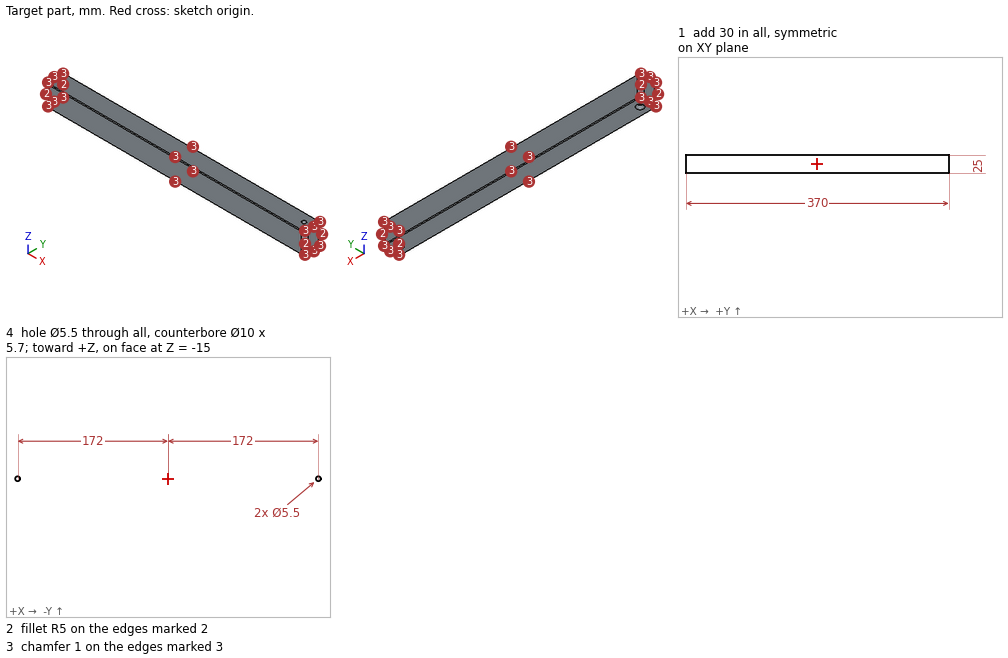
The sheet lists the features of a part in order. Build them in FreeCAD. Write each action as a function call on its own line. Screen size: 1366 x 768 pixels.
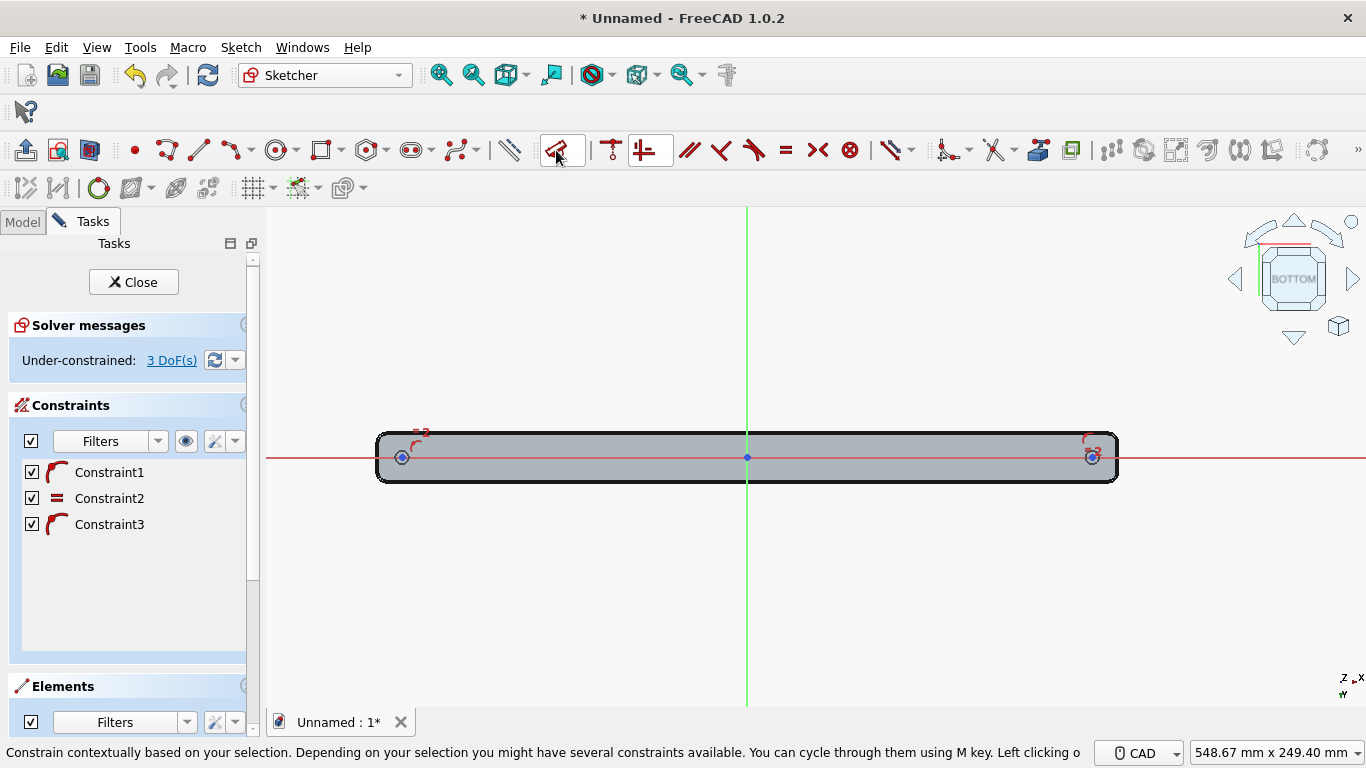
scroll(1099, 458, up, 7)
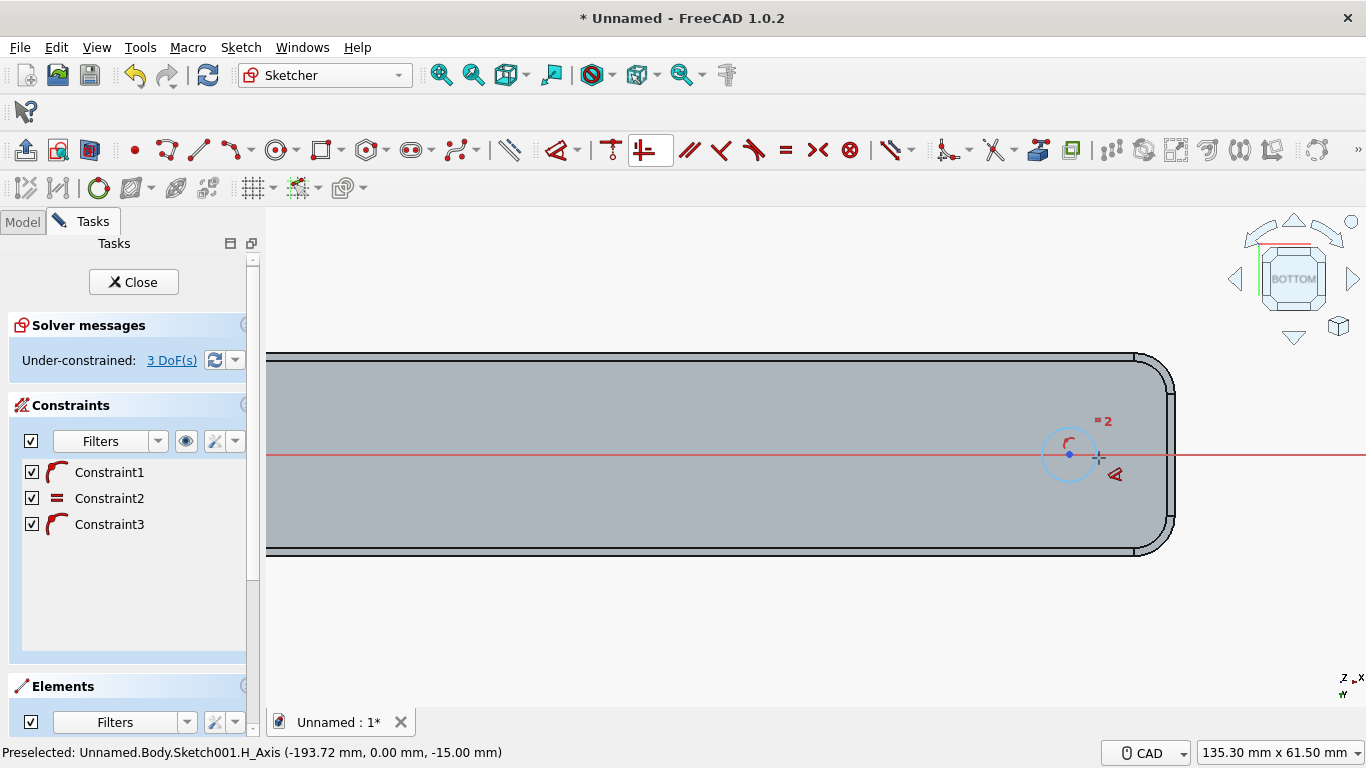
click(1096, 455)
click(1120, 483)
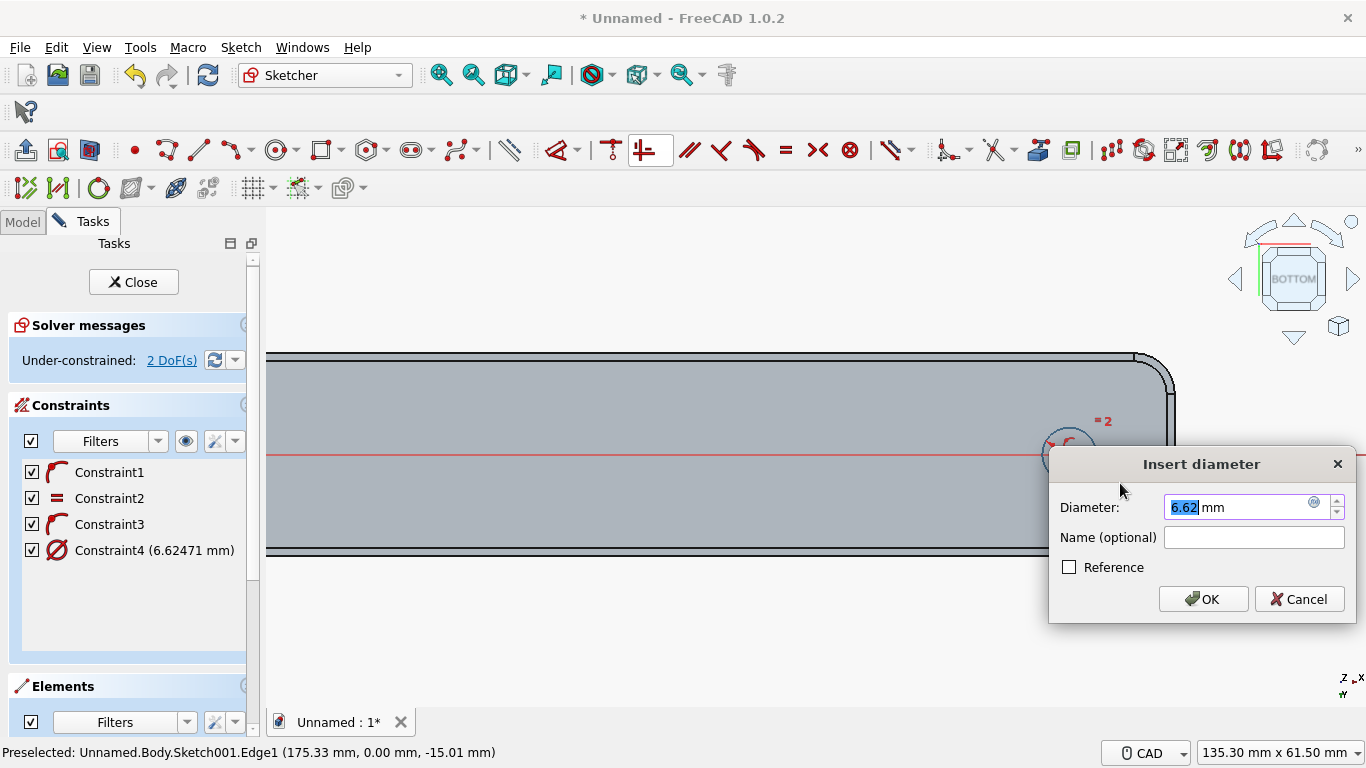
text(5.5)
key(Return)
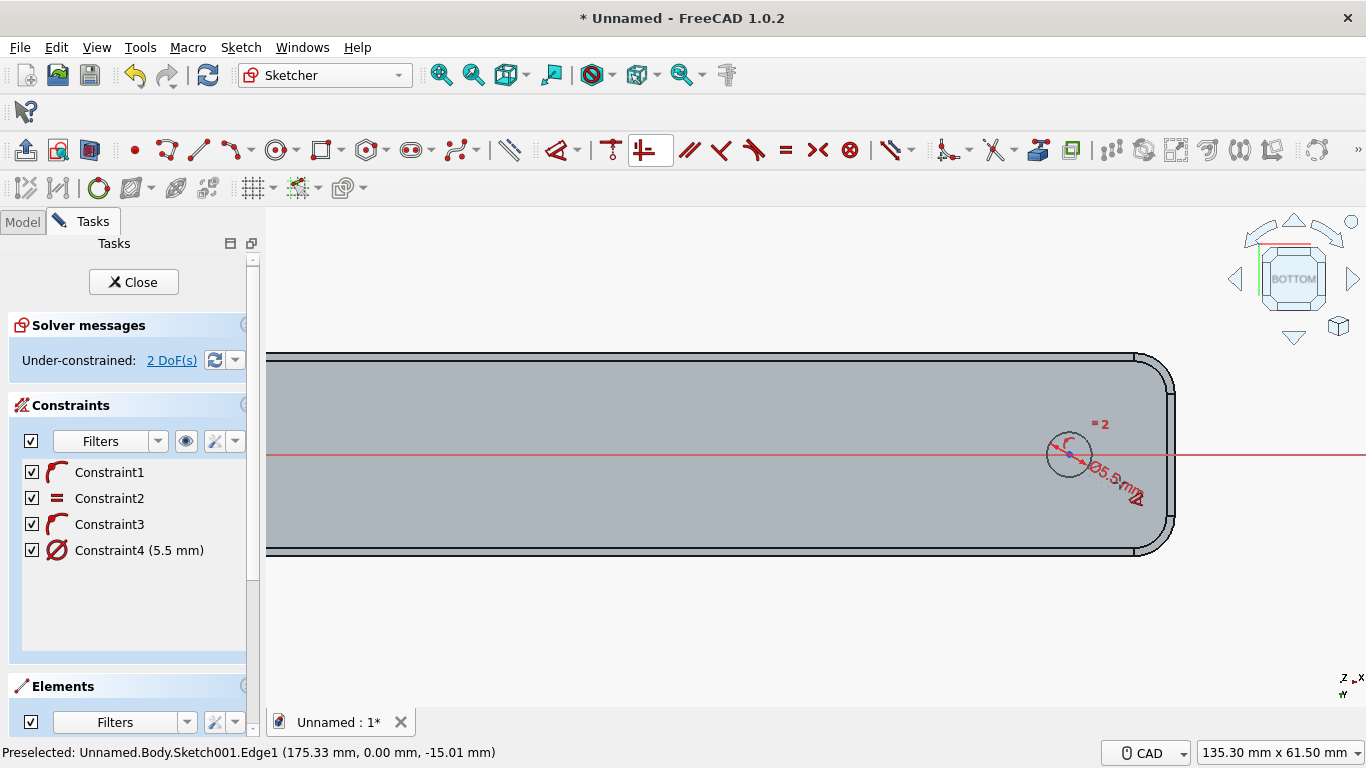
scroll(1100, 458, down, 7)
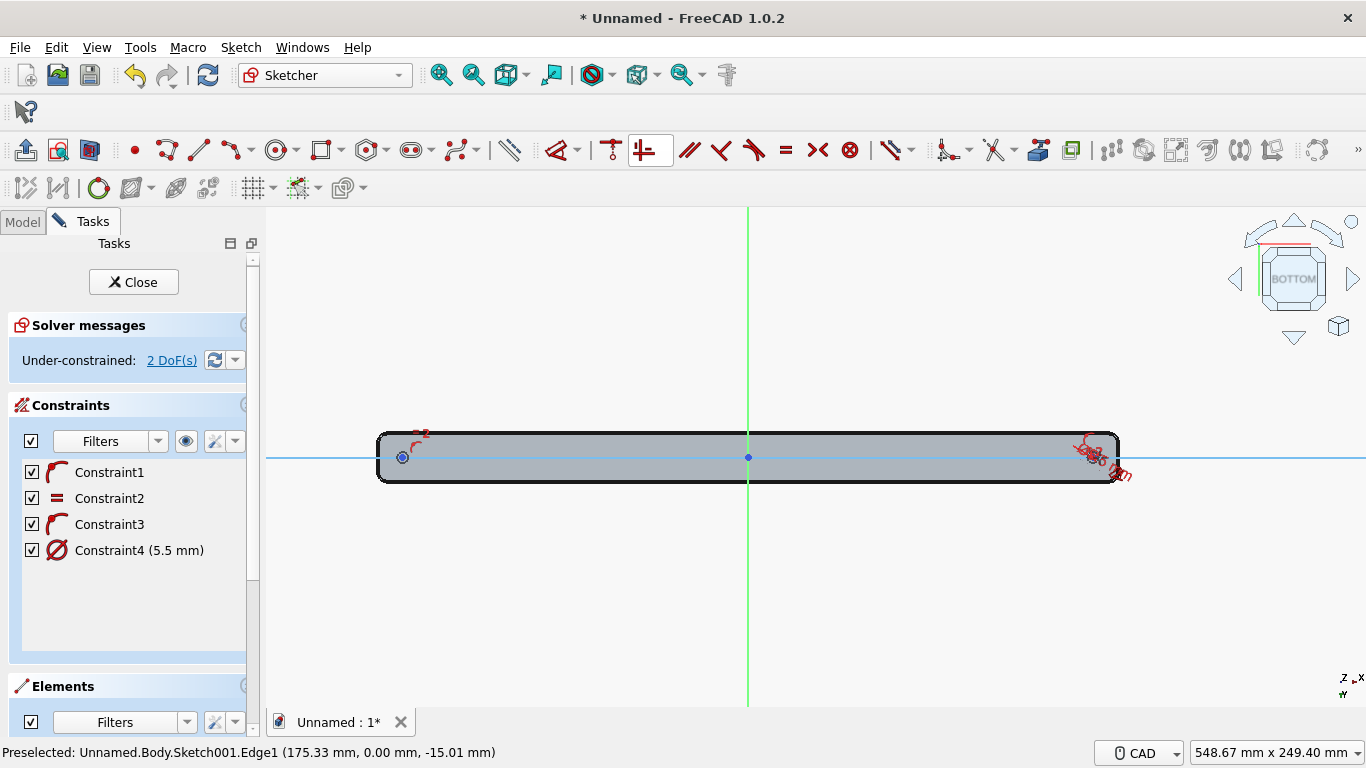
click(1093, 458)
click(921, 492)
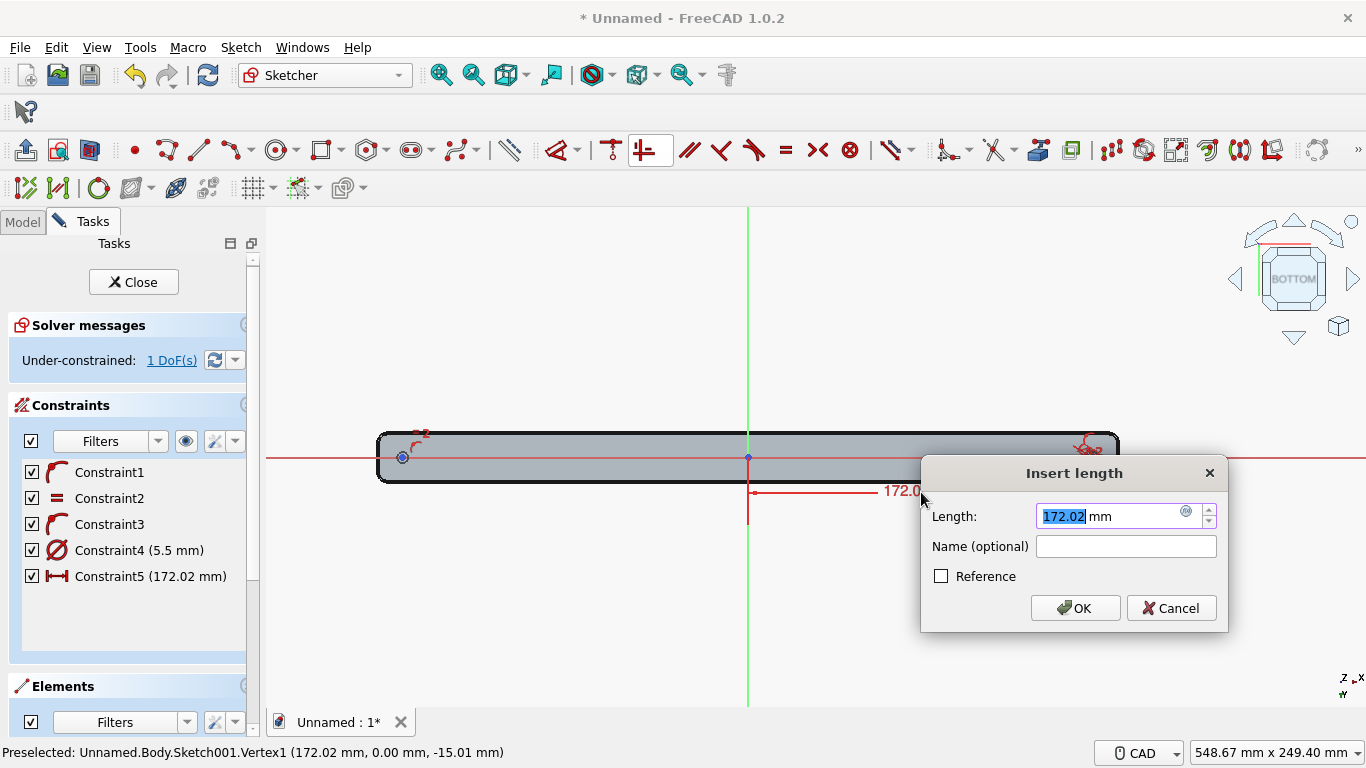
text(172)
key(Return)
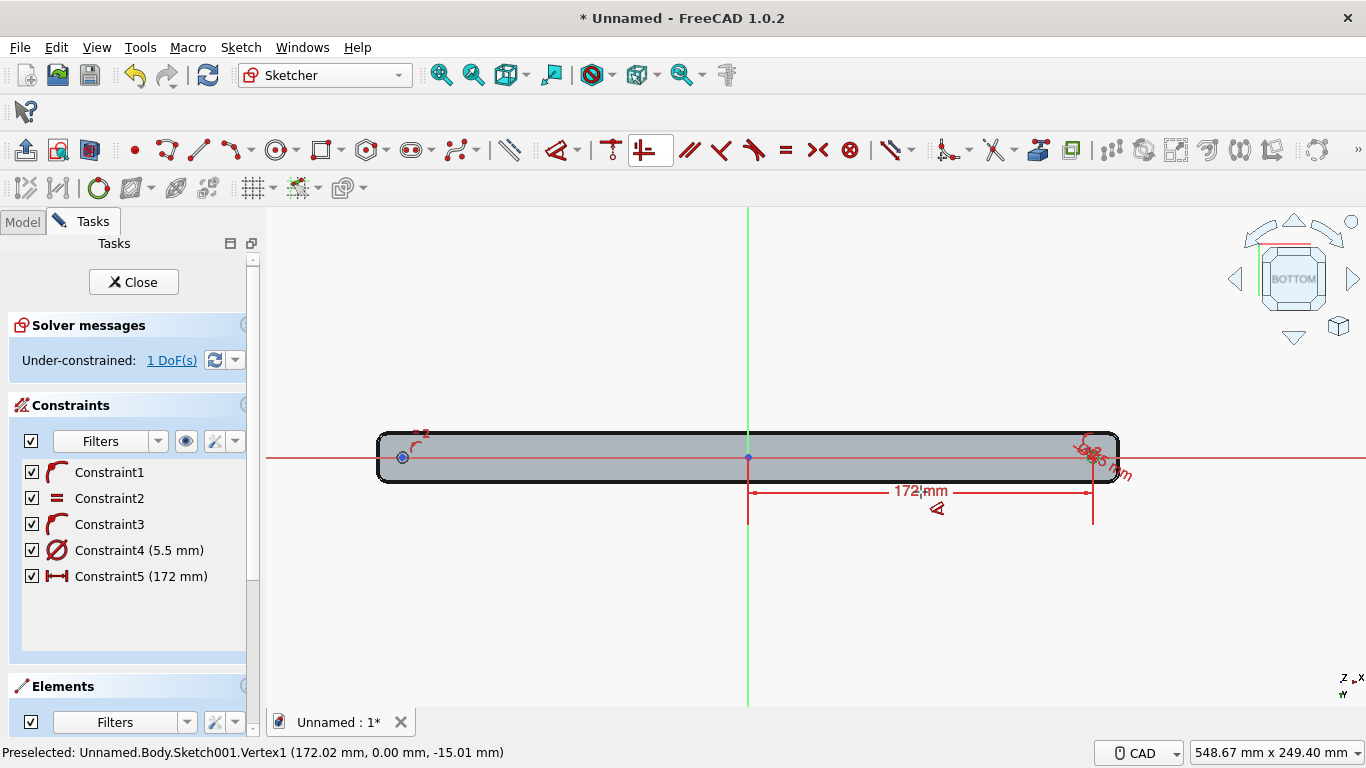
click(403, 458)
click(575, 492)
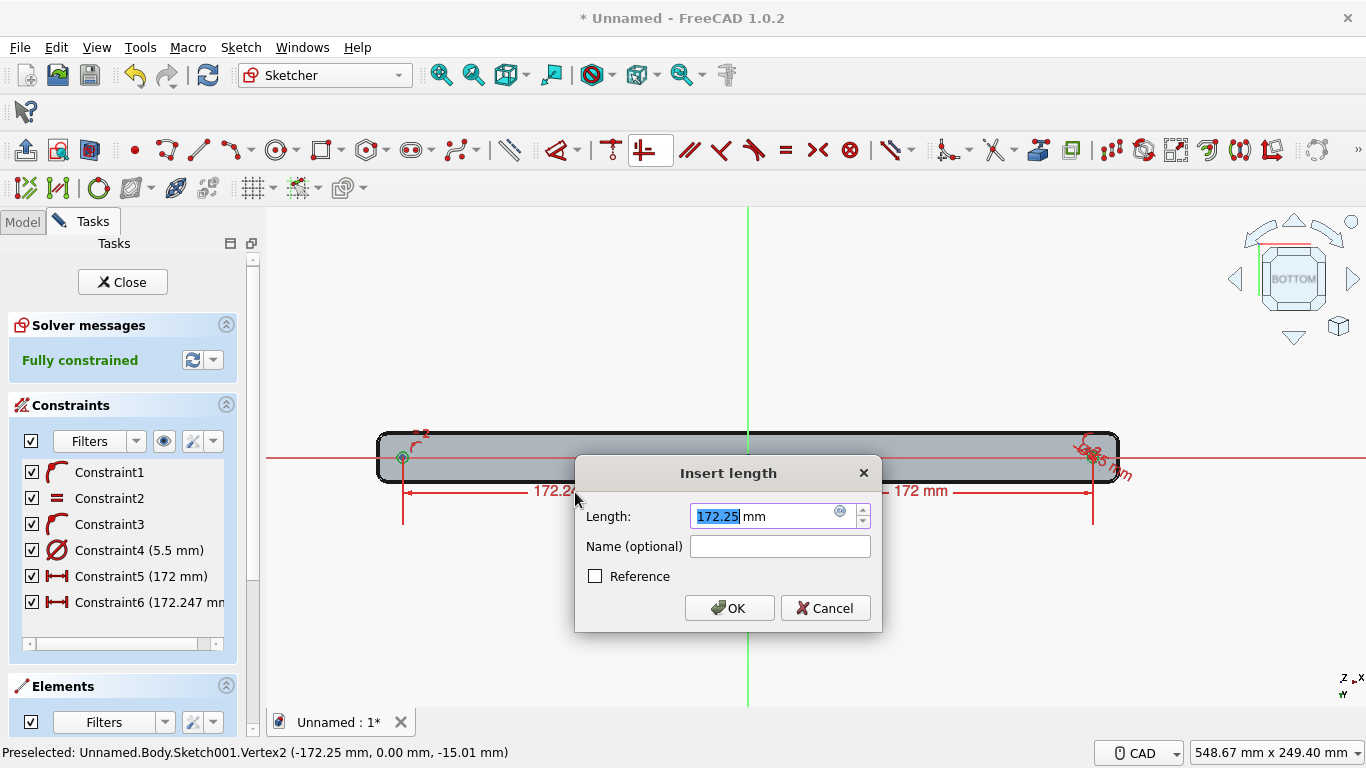
text(172)
key(Return)
key(Escape)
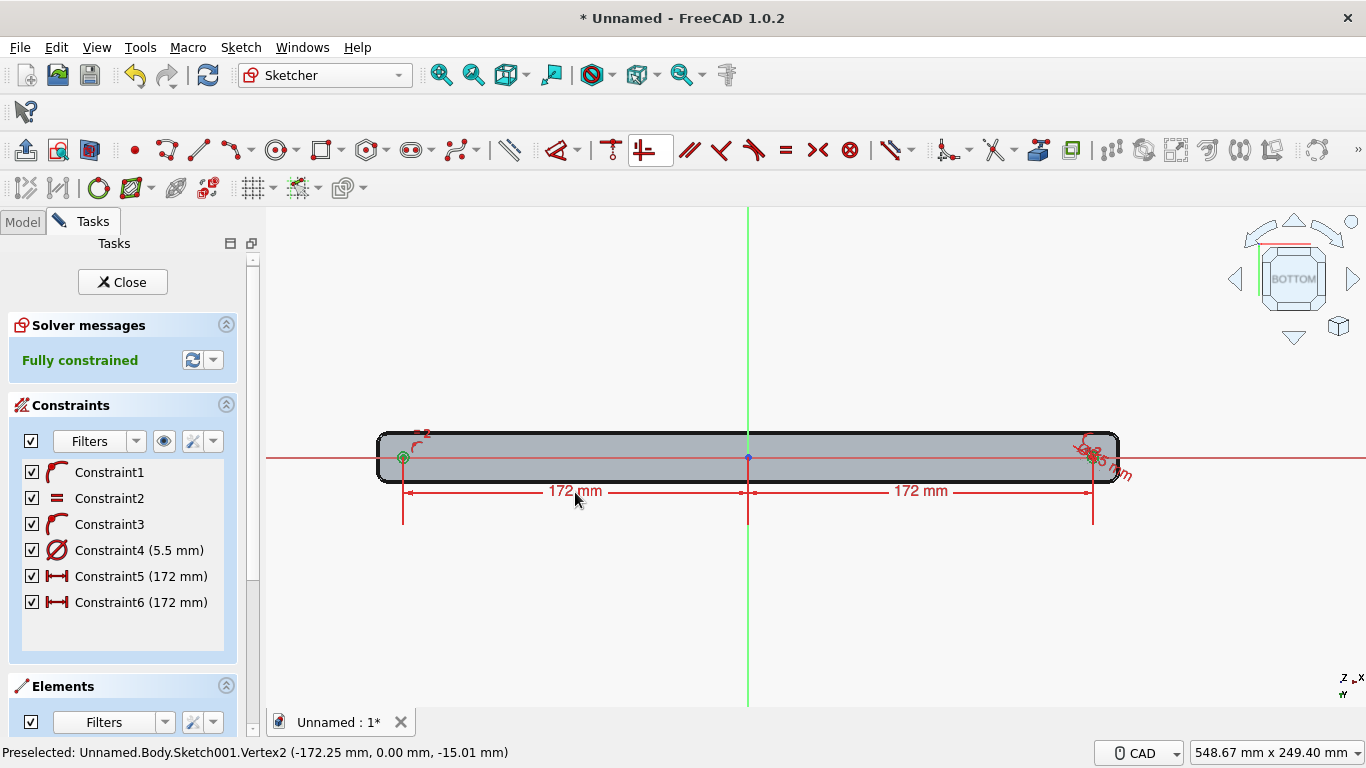
click(123, 282)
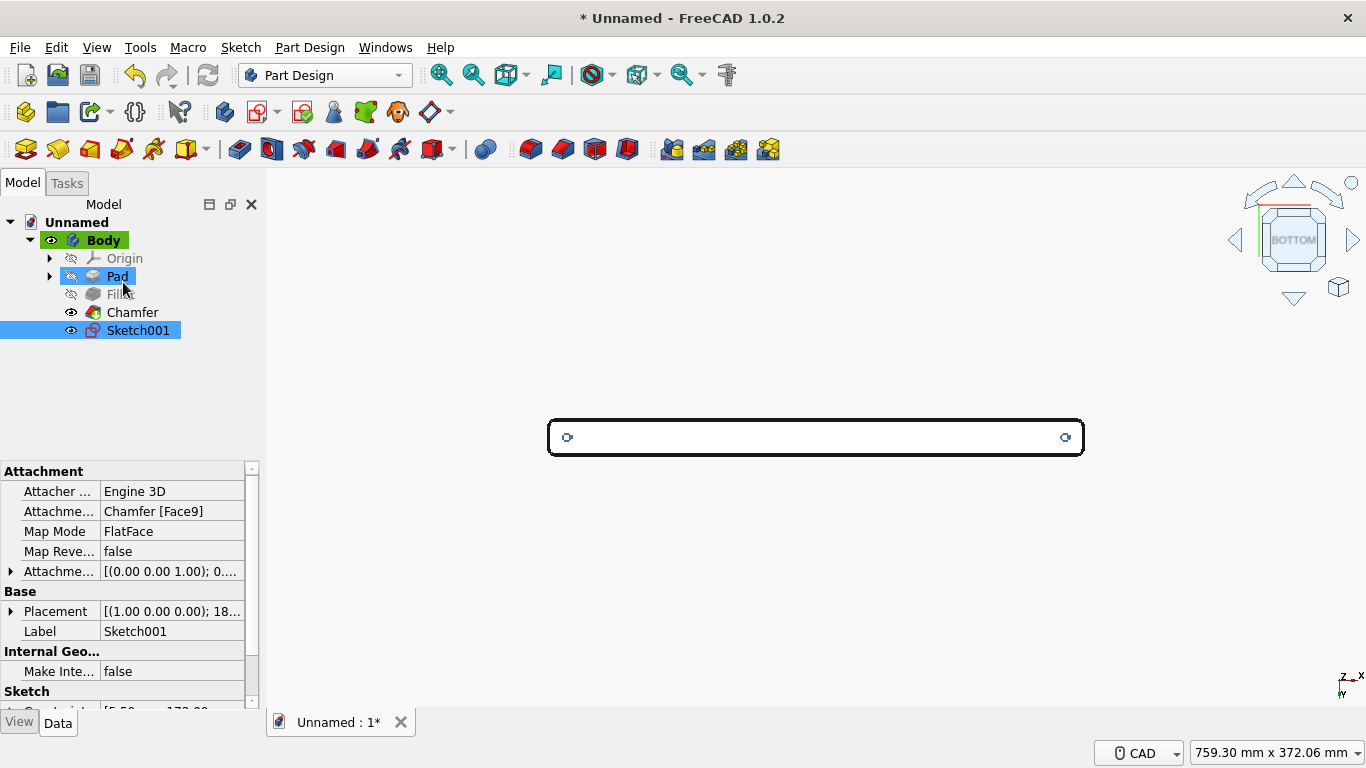
click(272, 150)